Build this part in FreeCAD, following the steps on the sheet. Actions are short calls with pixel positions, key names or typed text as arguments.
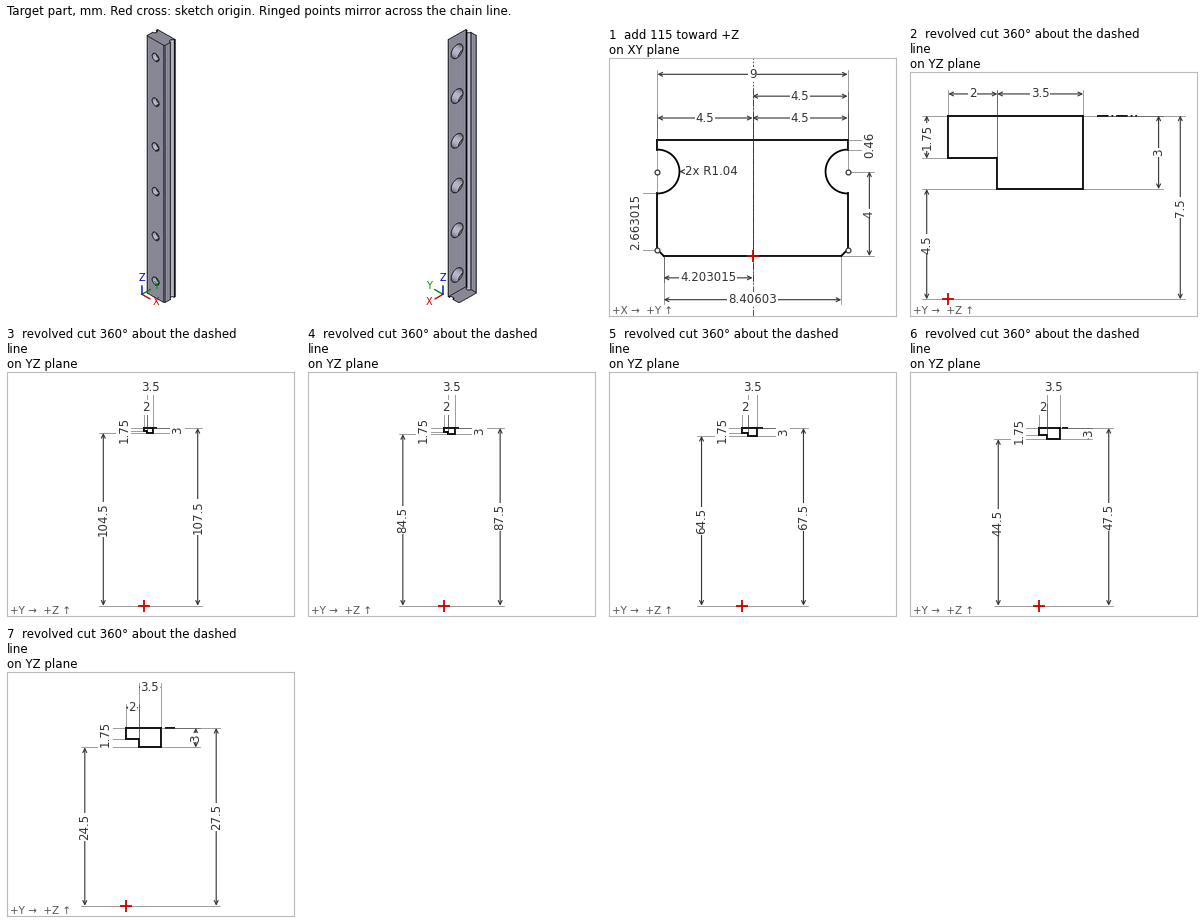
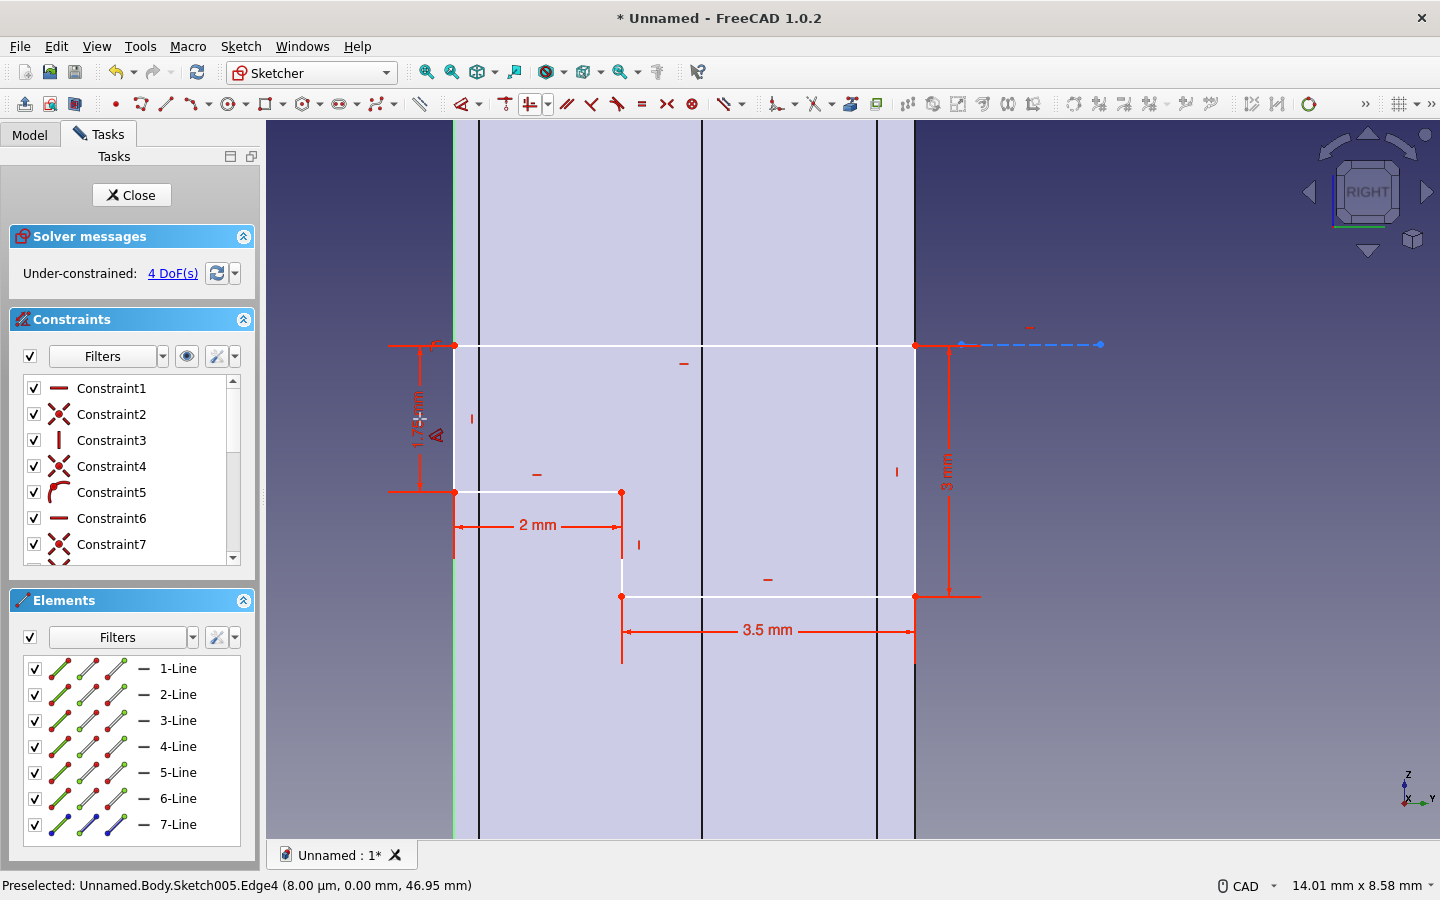
click(622, 597)
click(420, 704)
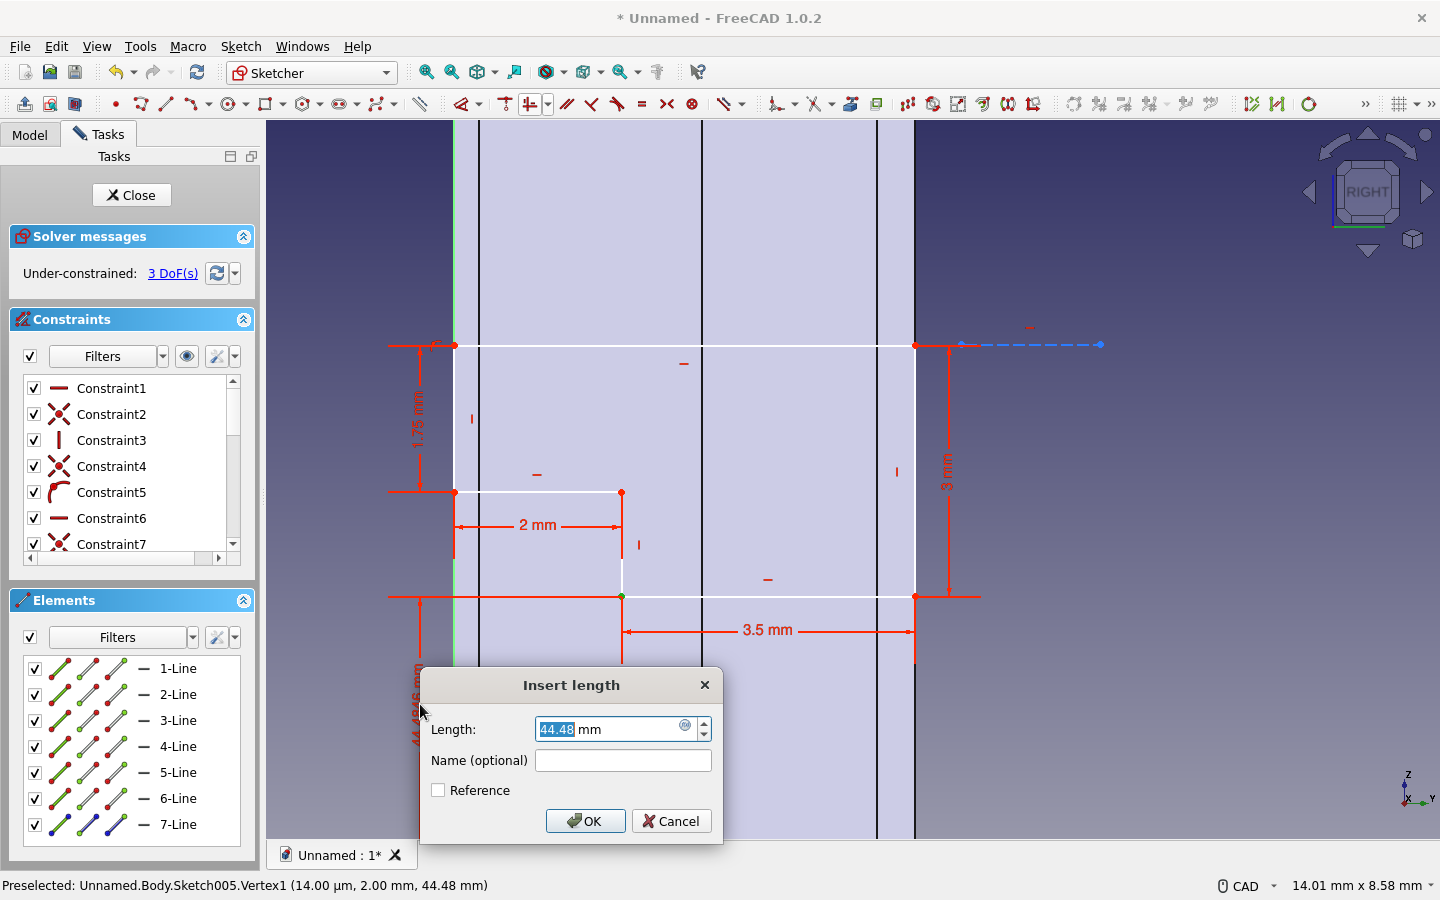
text(44.5)
key(Return)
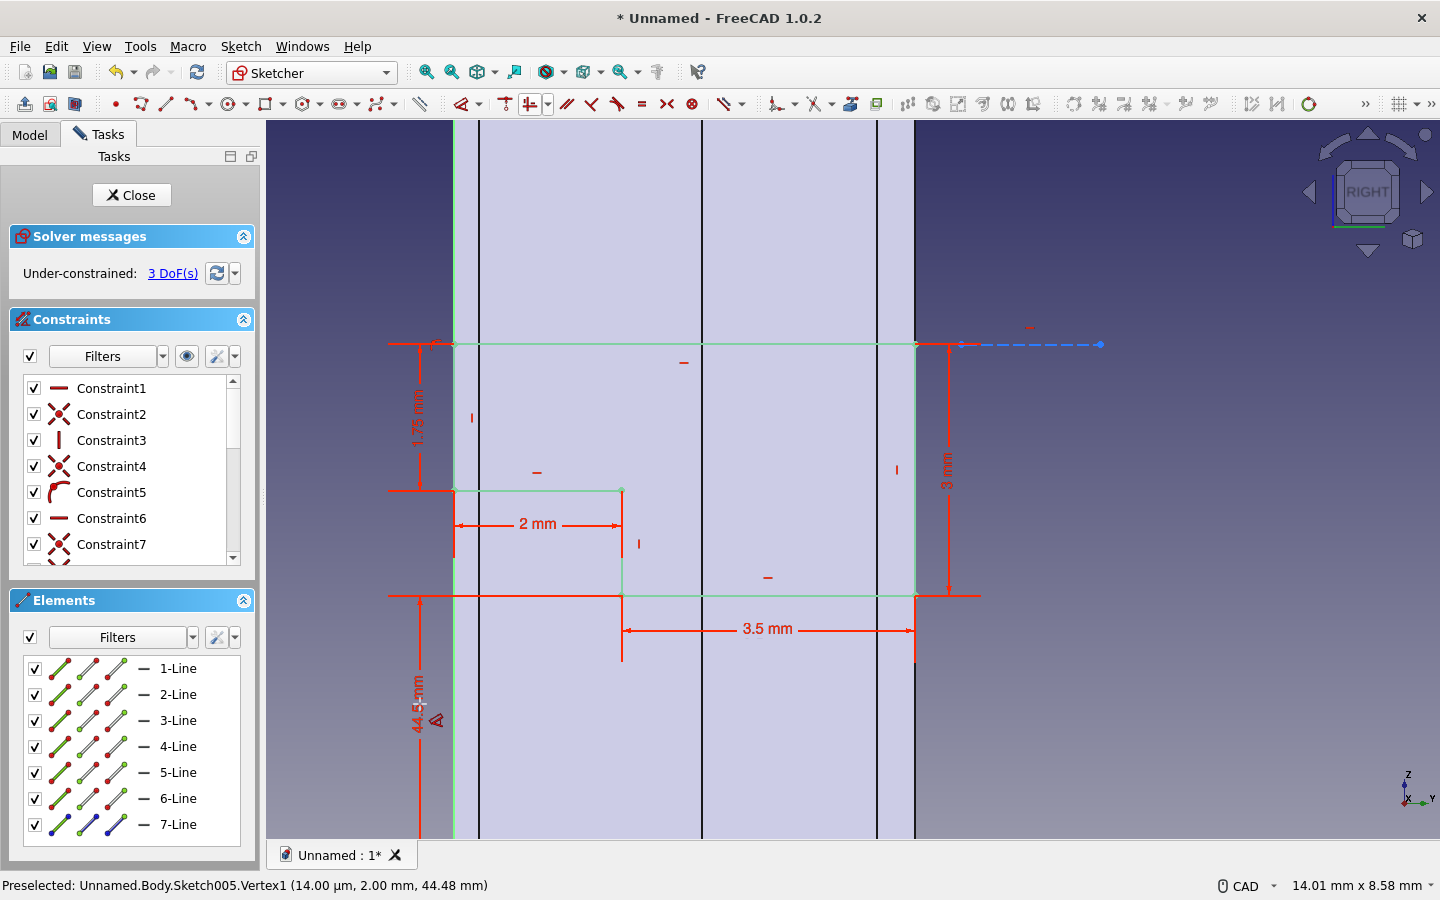
click(961, 345)
click(420, 578)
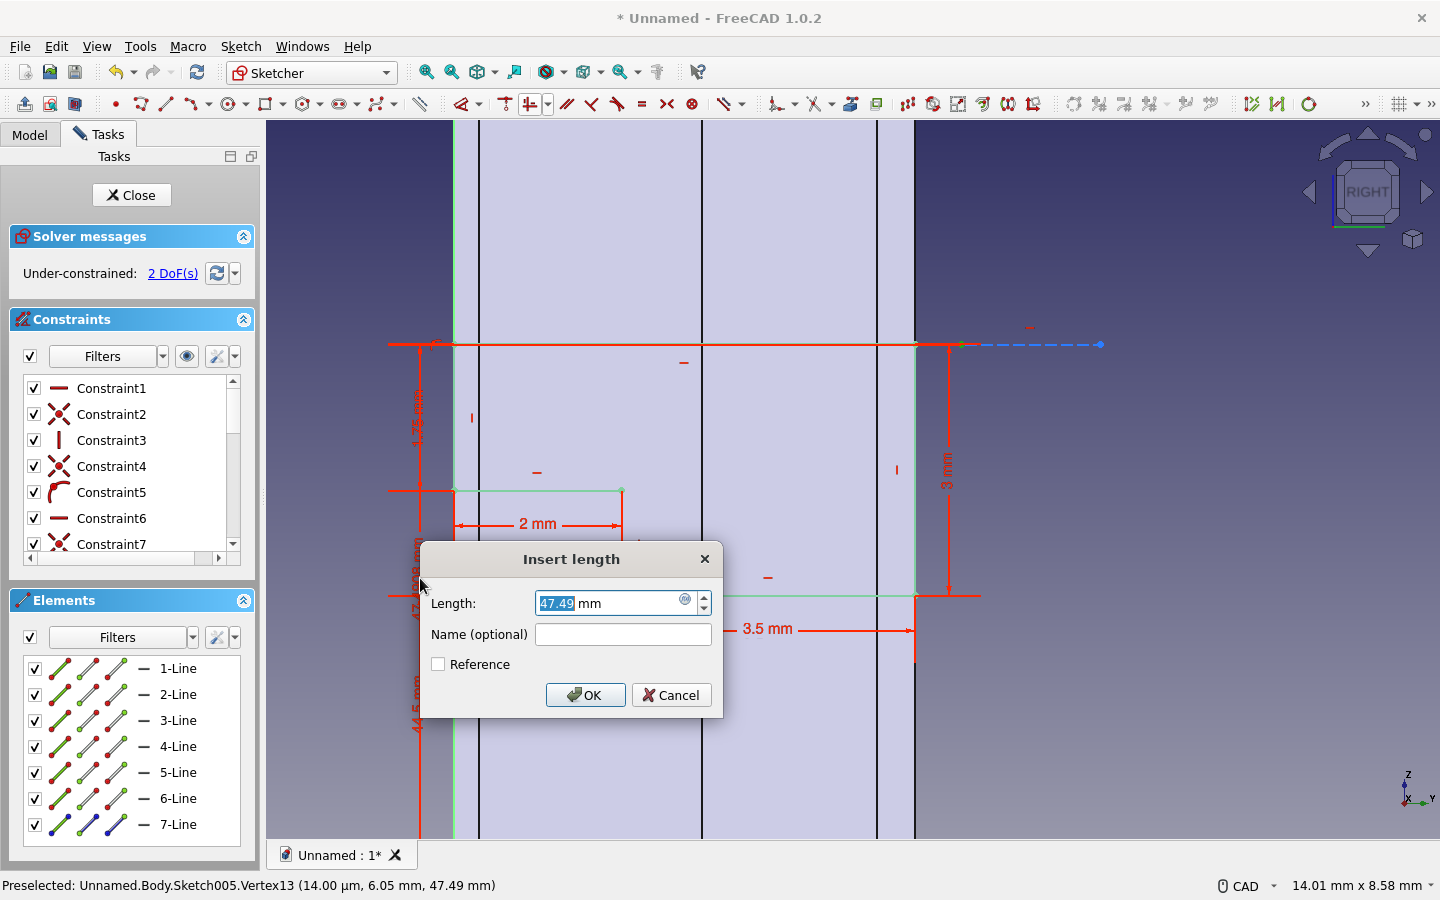
text(47.5)
key(Return)
key(Escape)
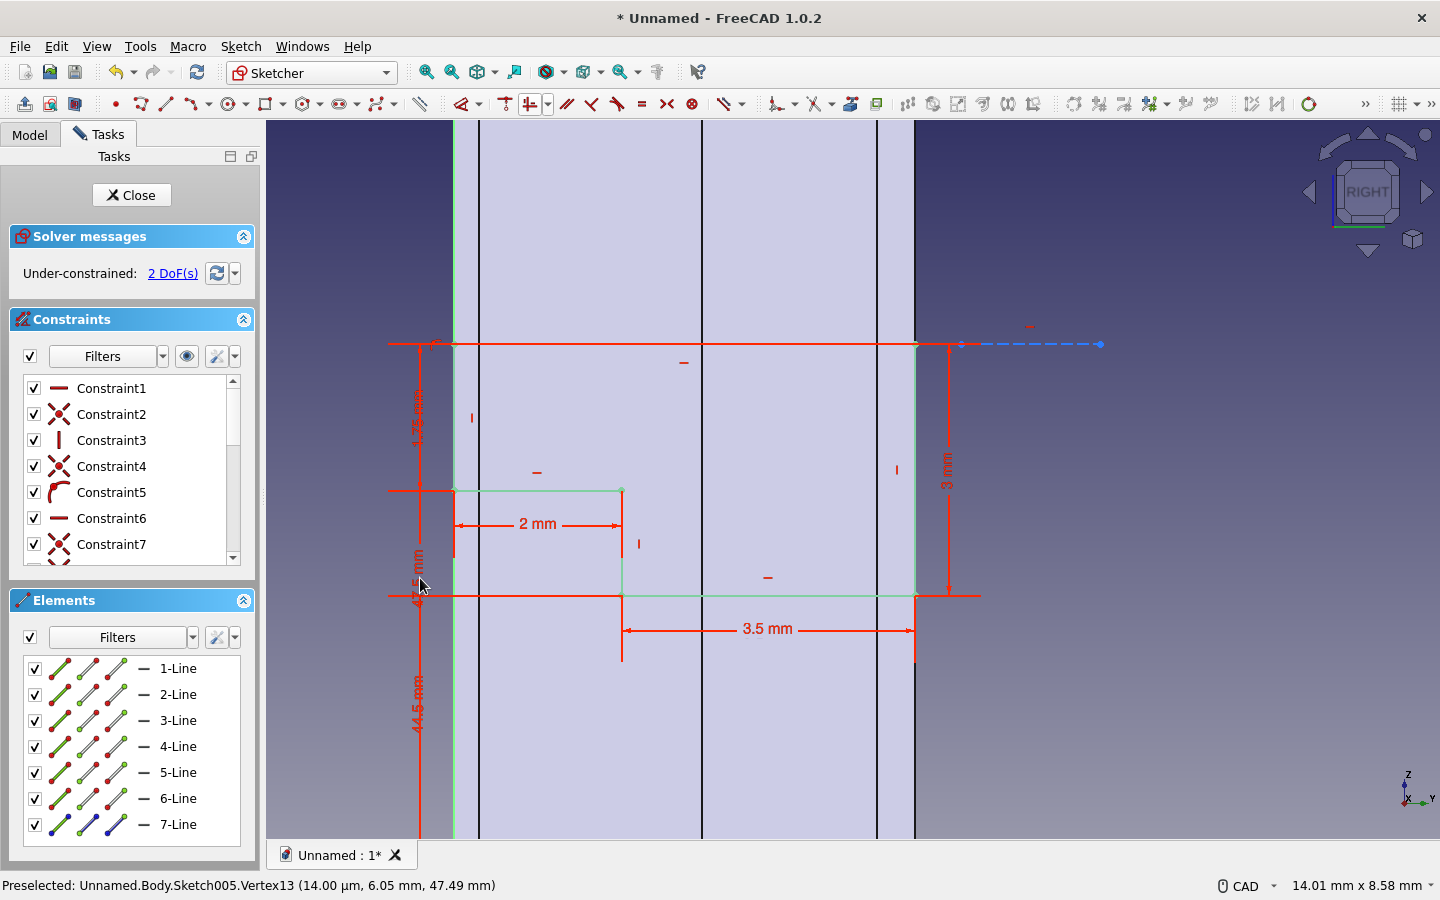
click(132, 195)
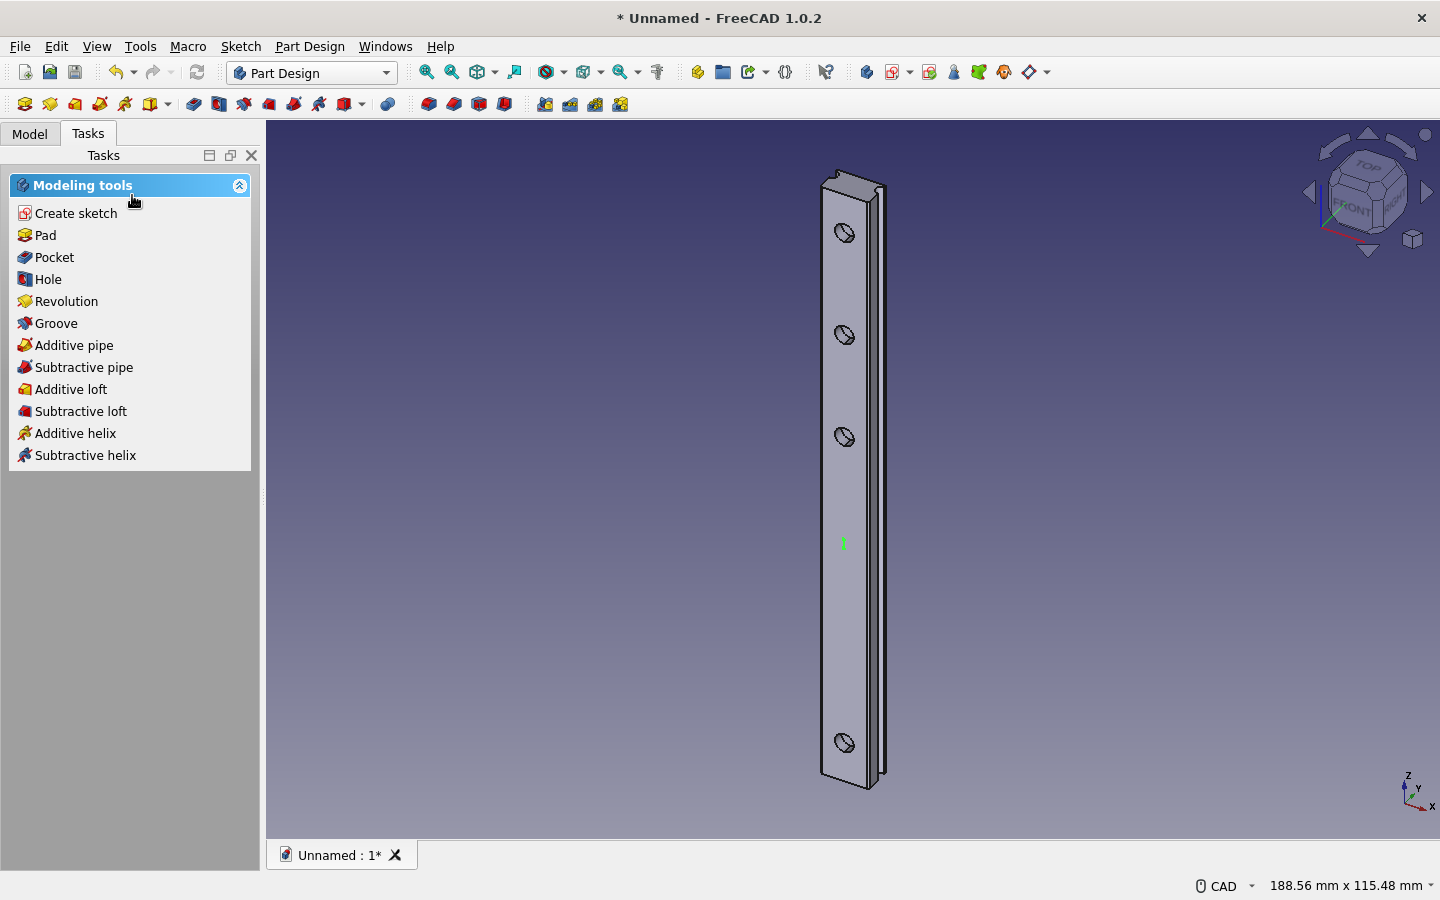
click(244, 104)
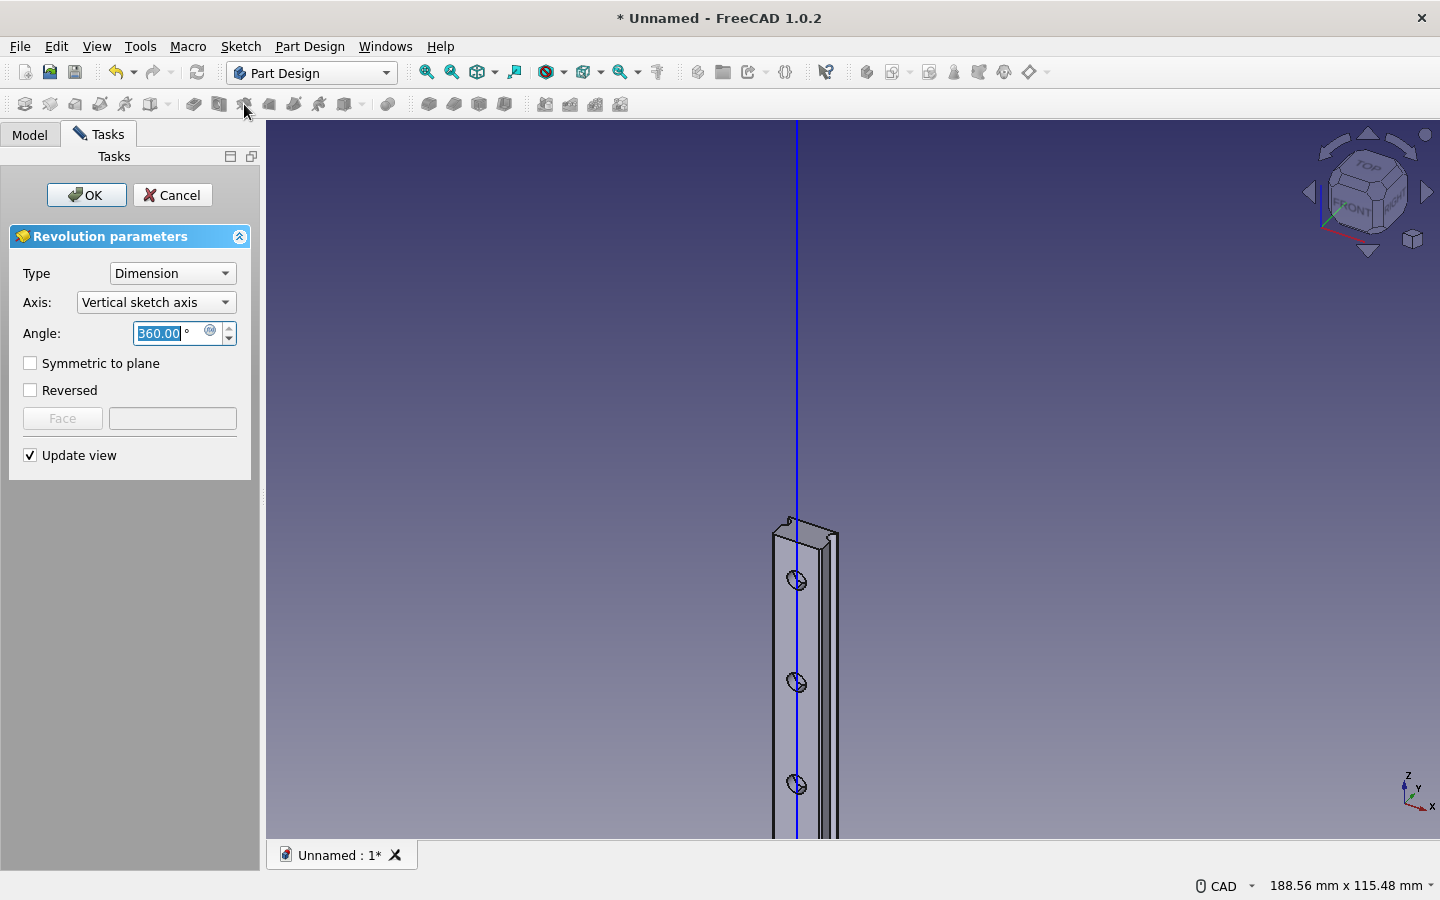
click(157, 302)